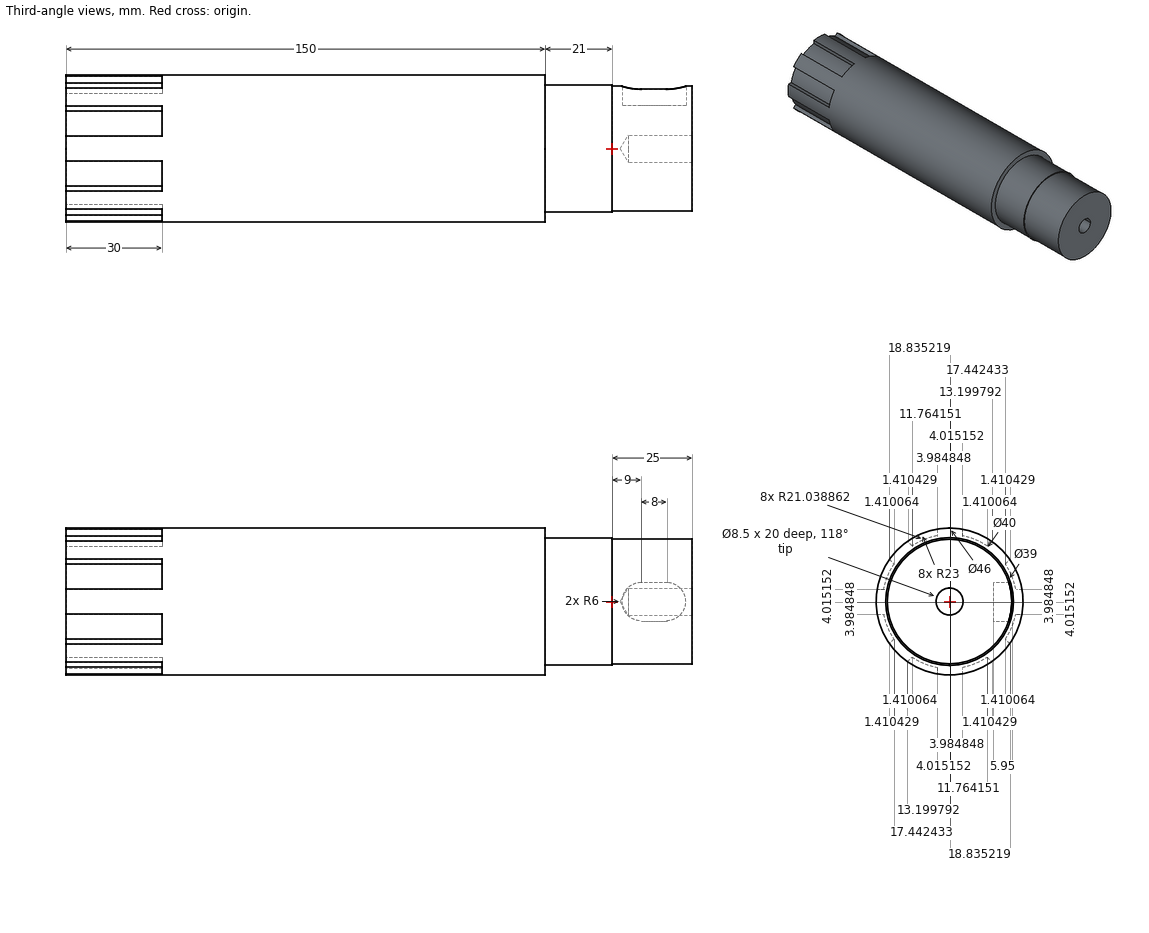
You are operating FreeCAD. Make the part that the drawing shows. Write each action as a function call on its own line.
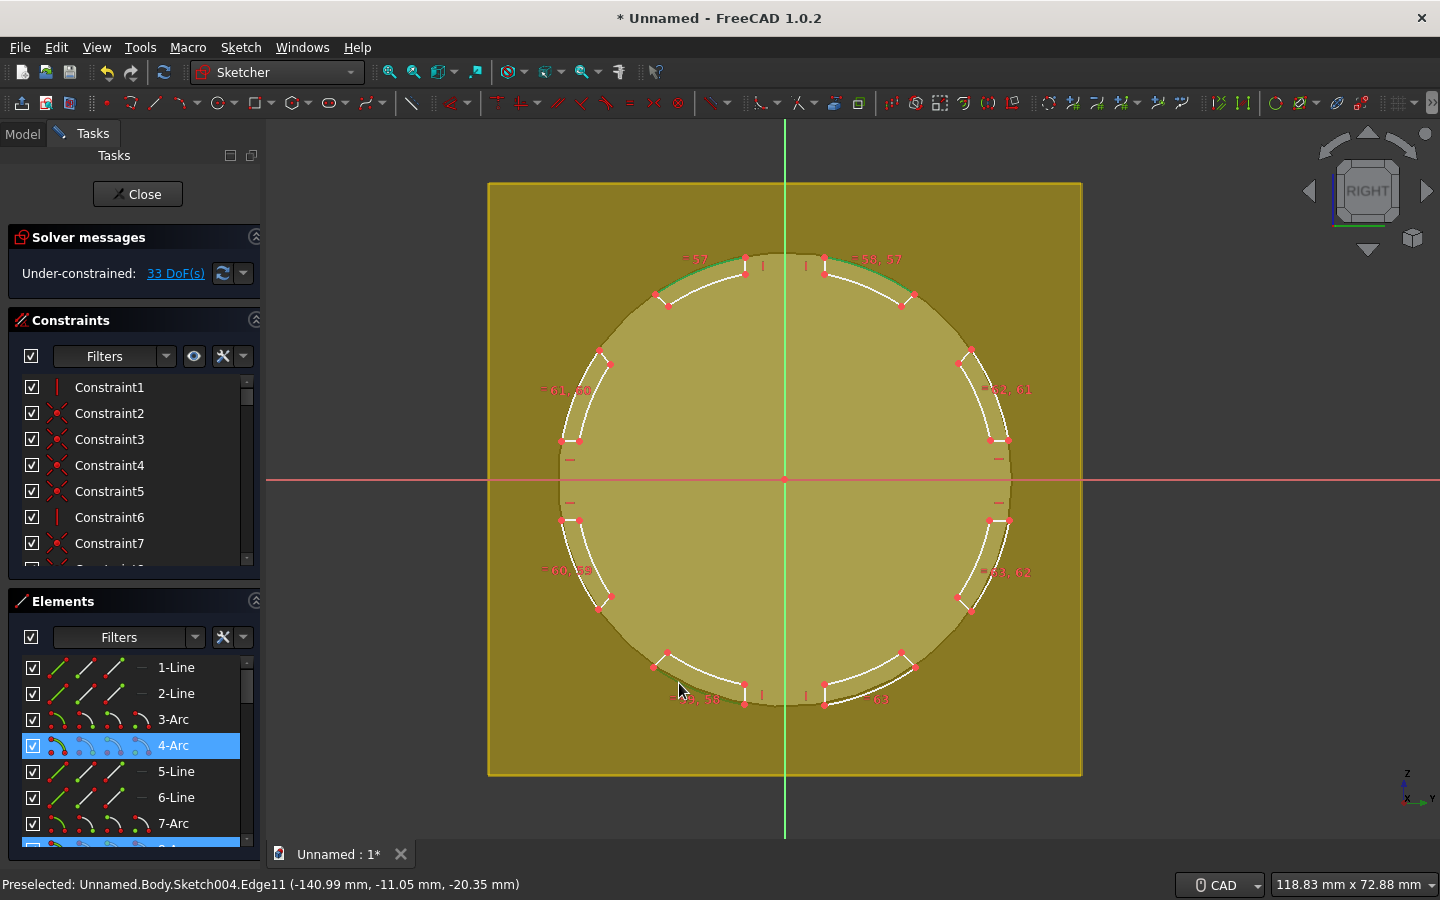
click(568, 549)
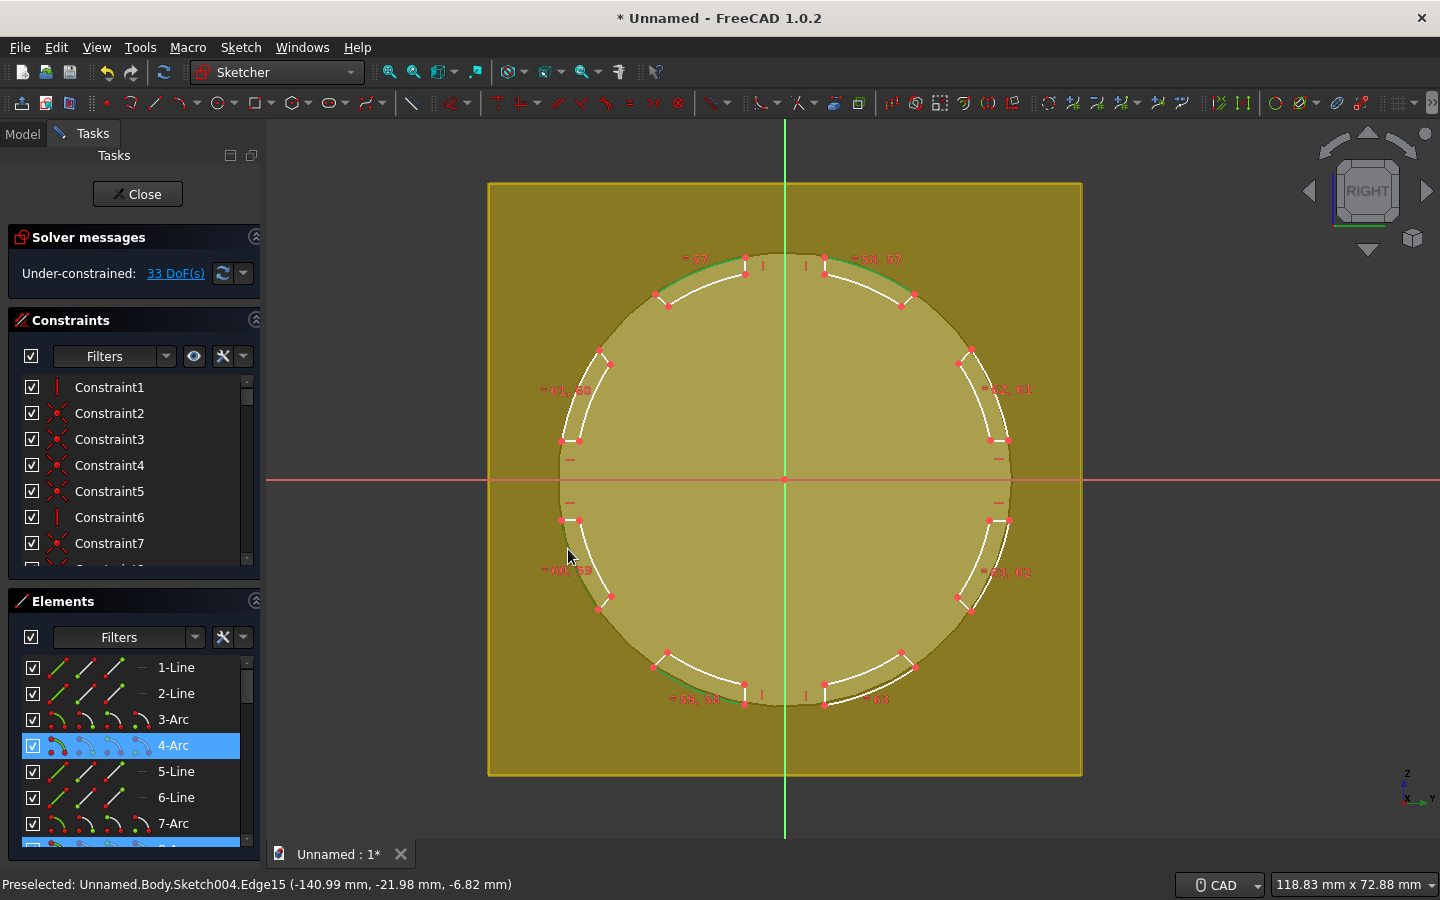
click(584, 376)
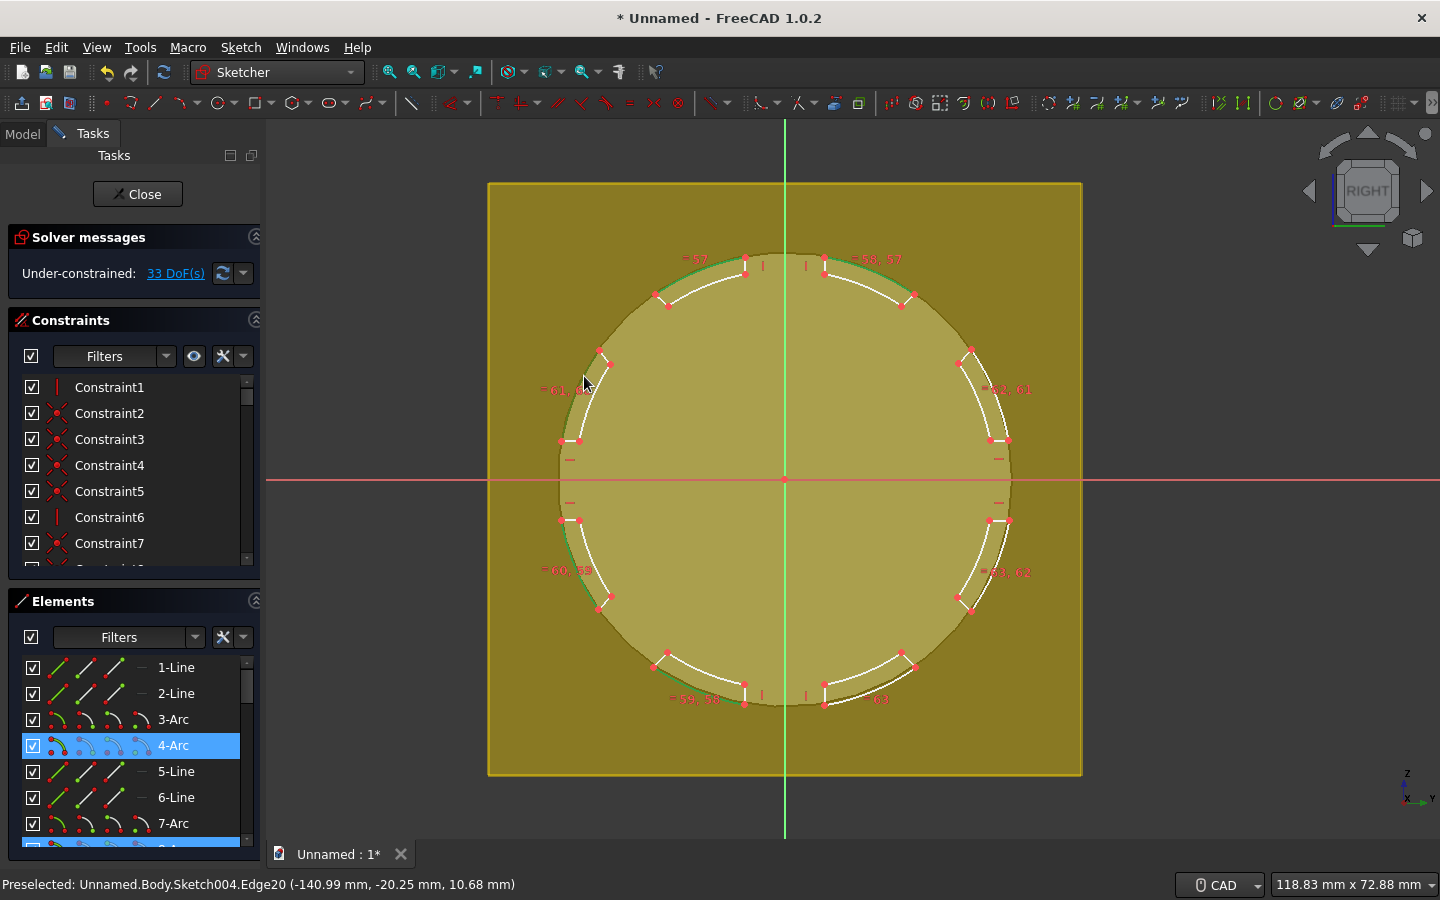
click(1002, 412)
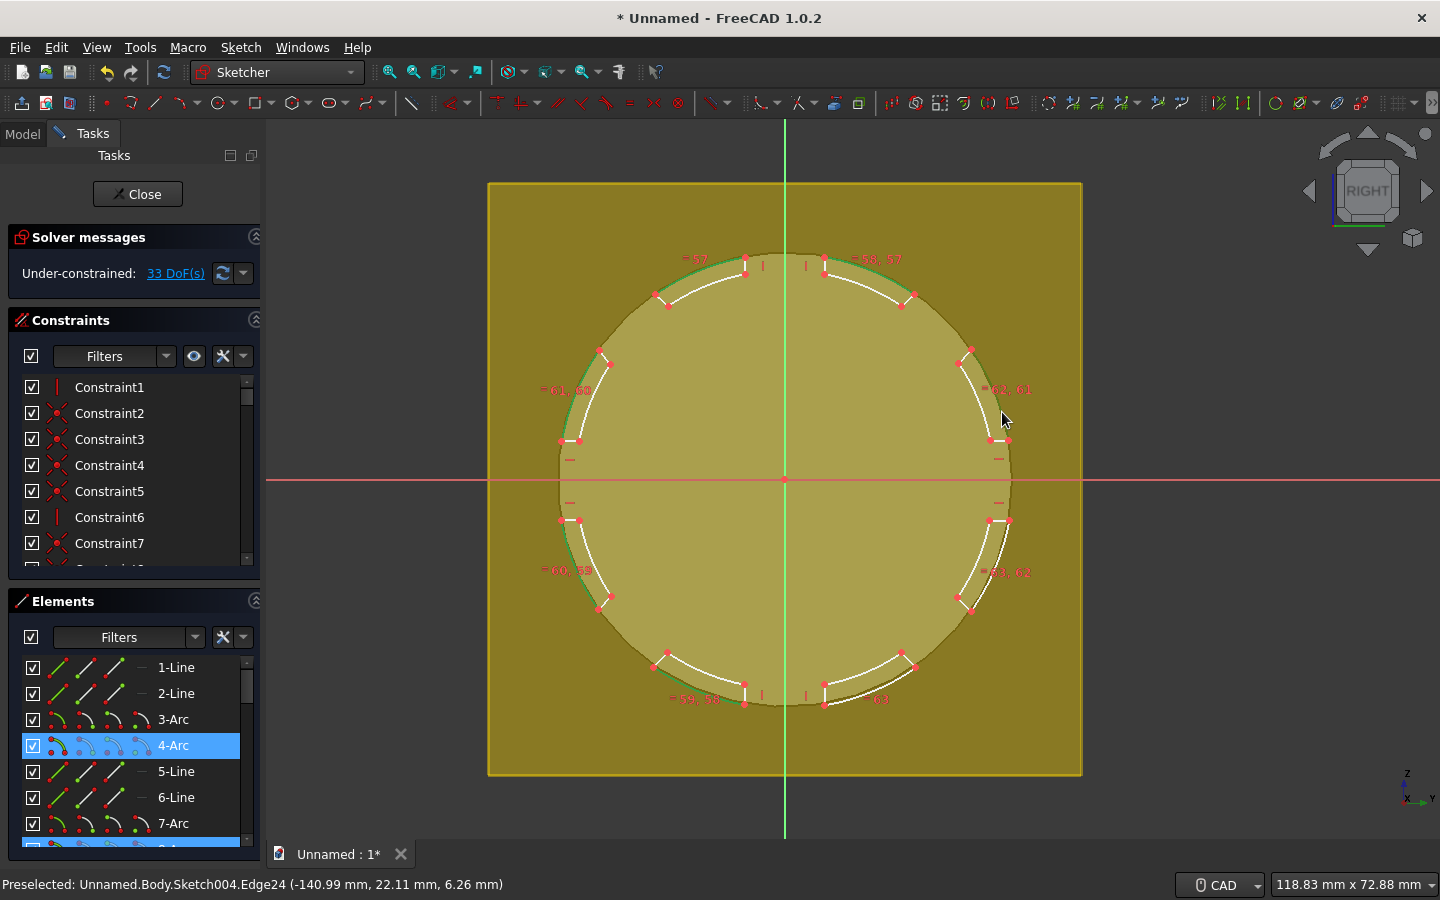
click(987, 586)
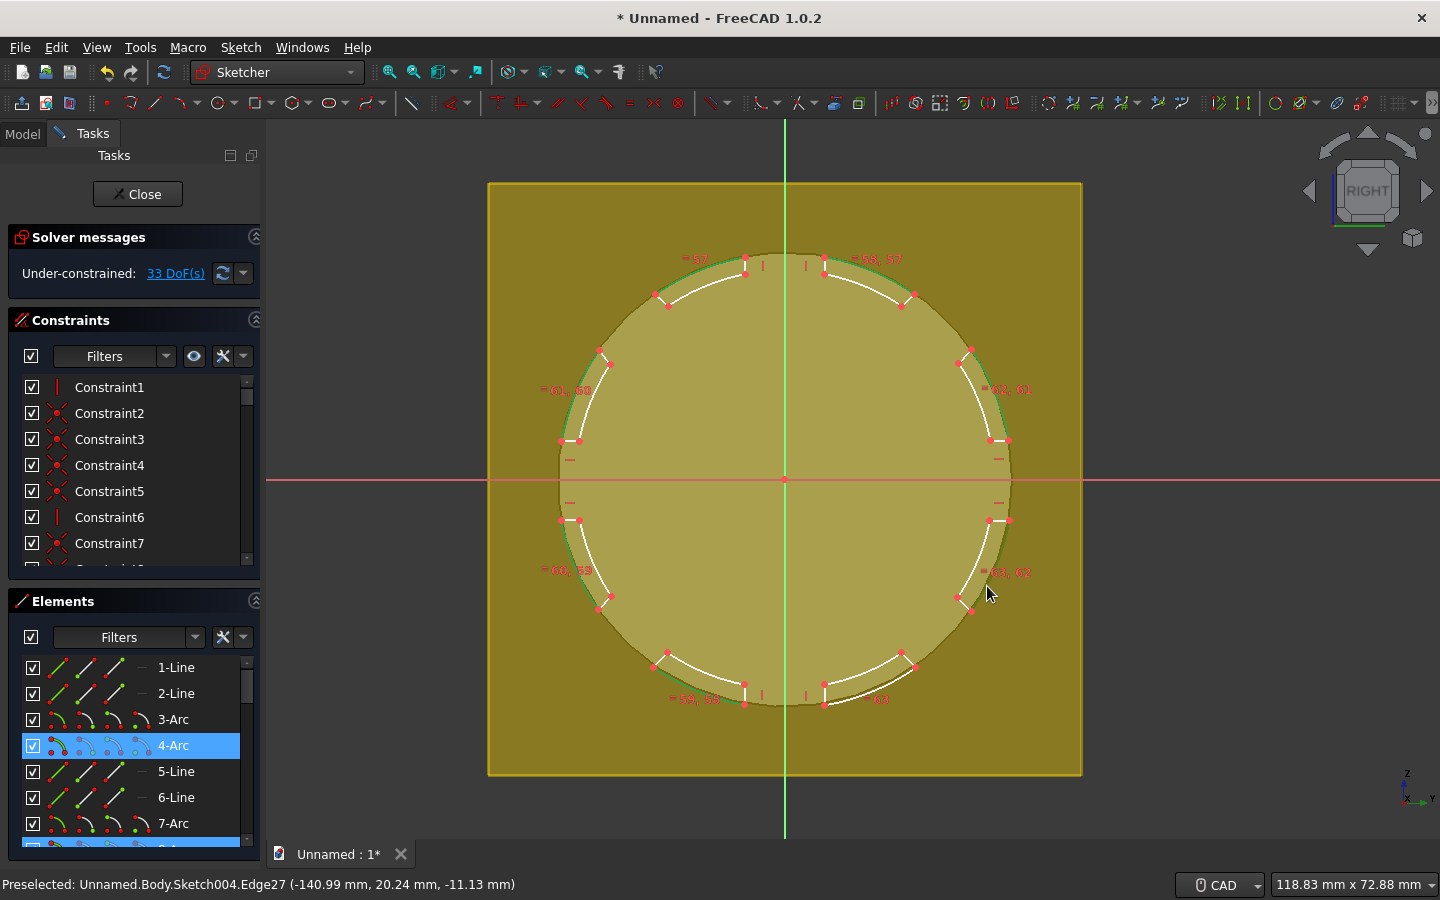
click(854, 698)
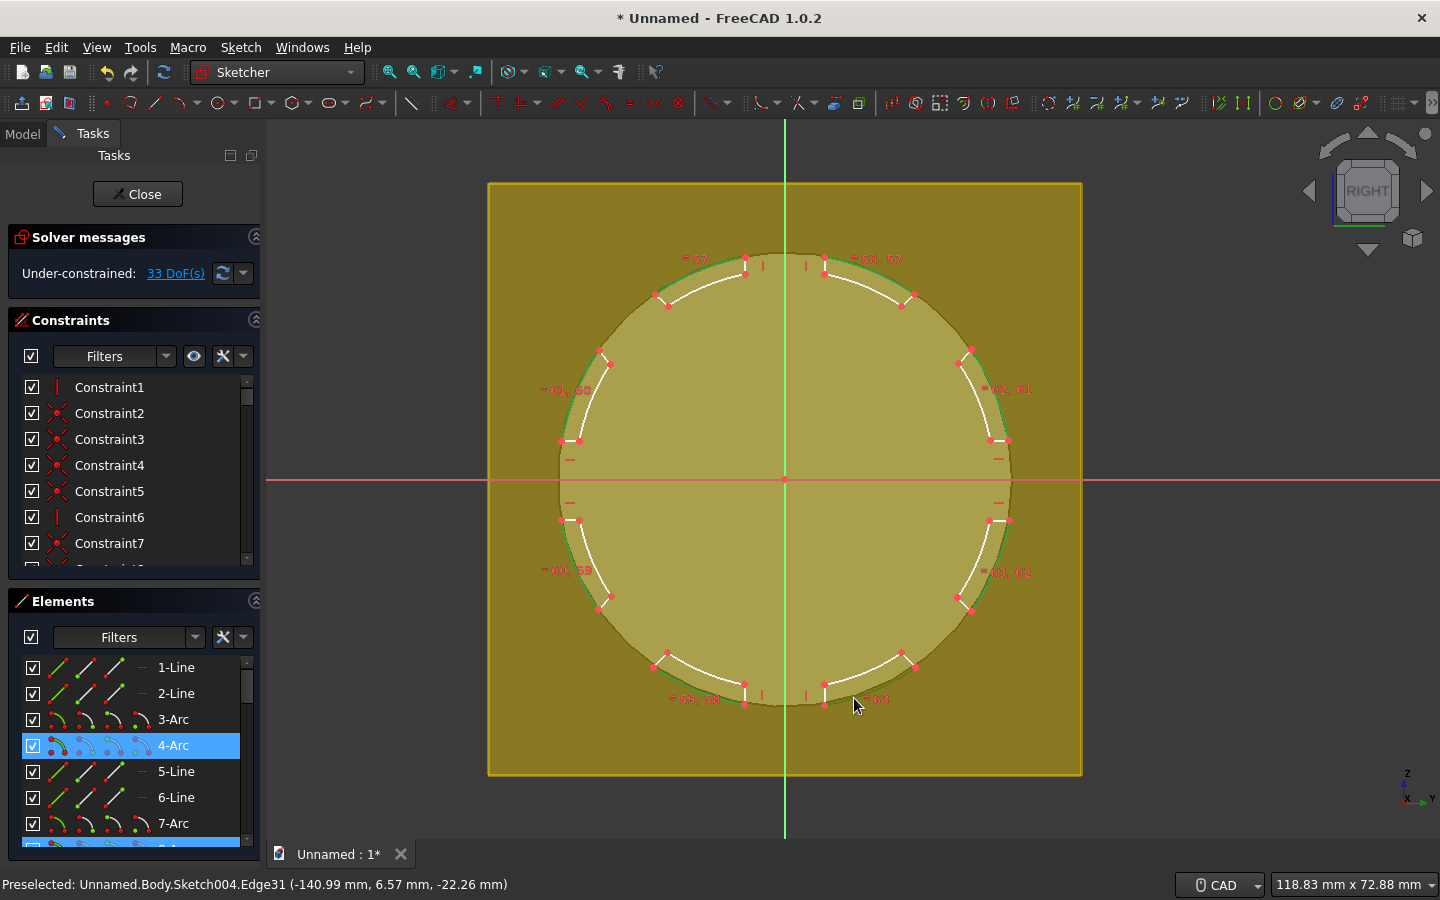
click(630, 104)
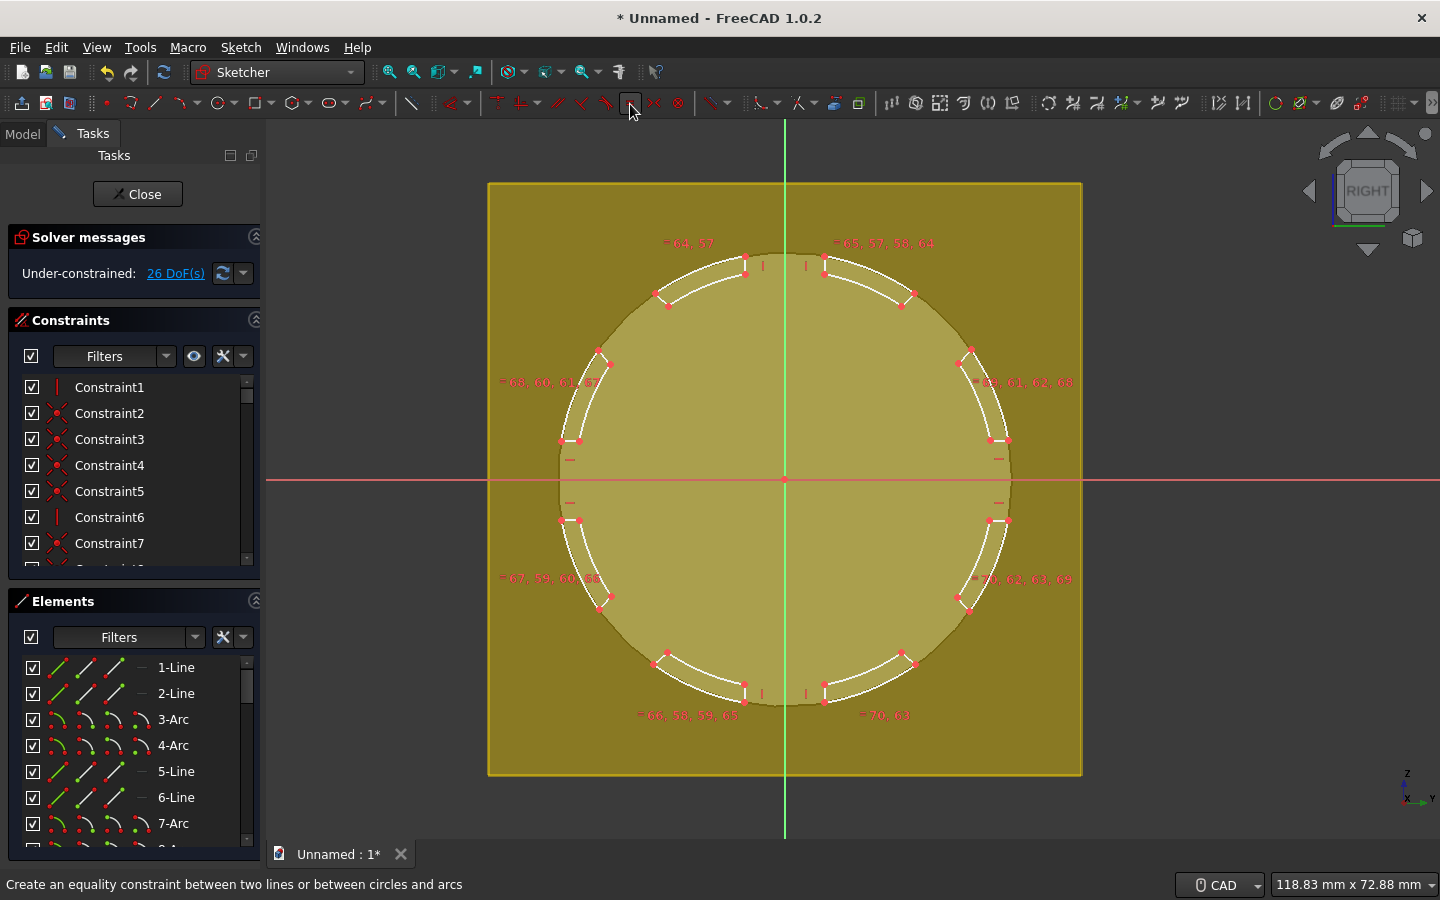
click(450, 104)